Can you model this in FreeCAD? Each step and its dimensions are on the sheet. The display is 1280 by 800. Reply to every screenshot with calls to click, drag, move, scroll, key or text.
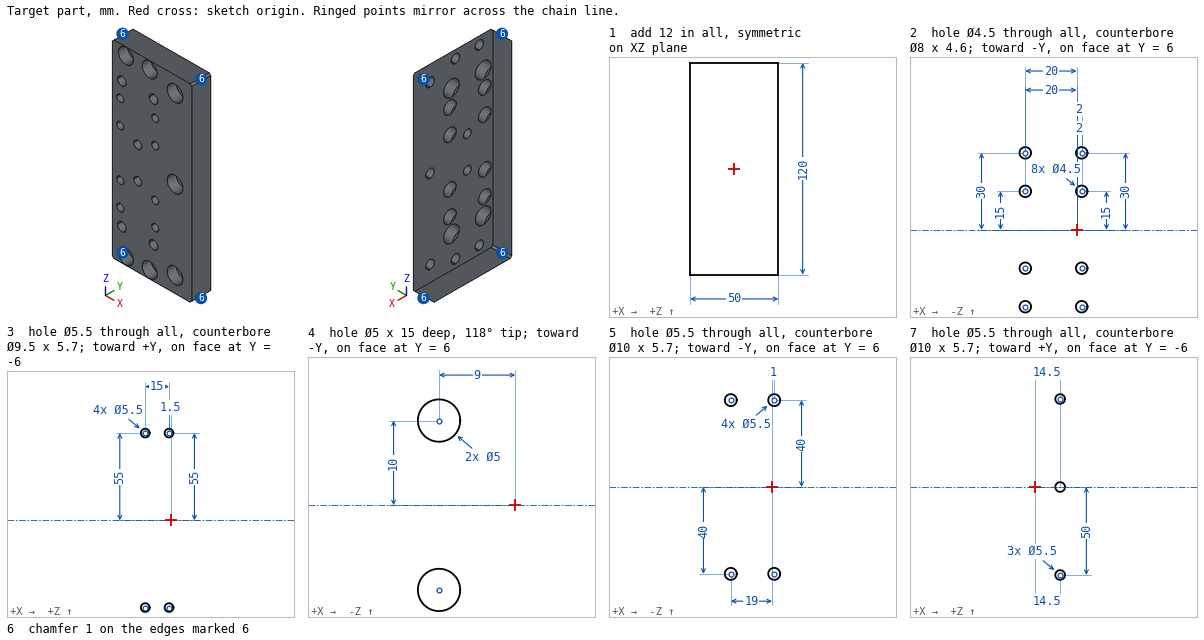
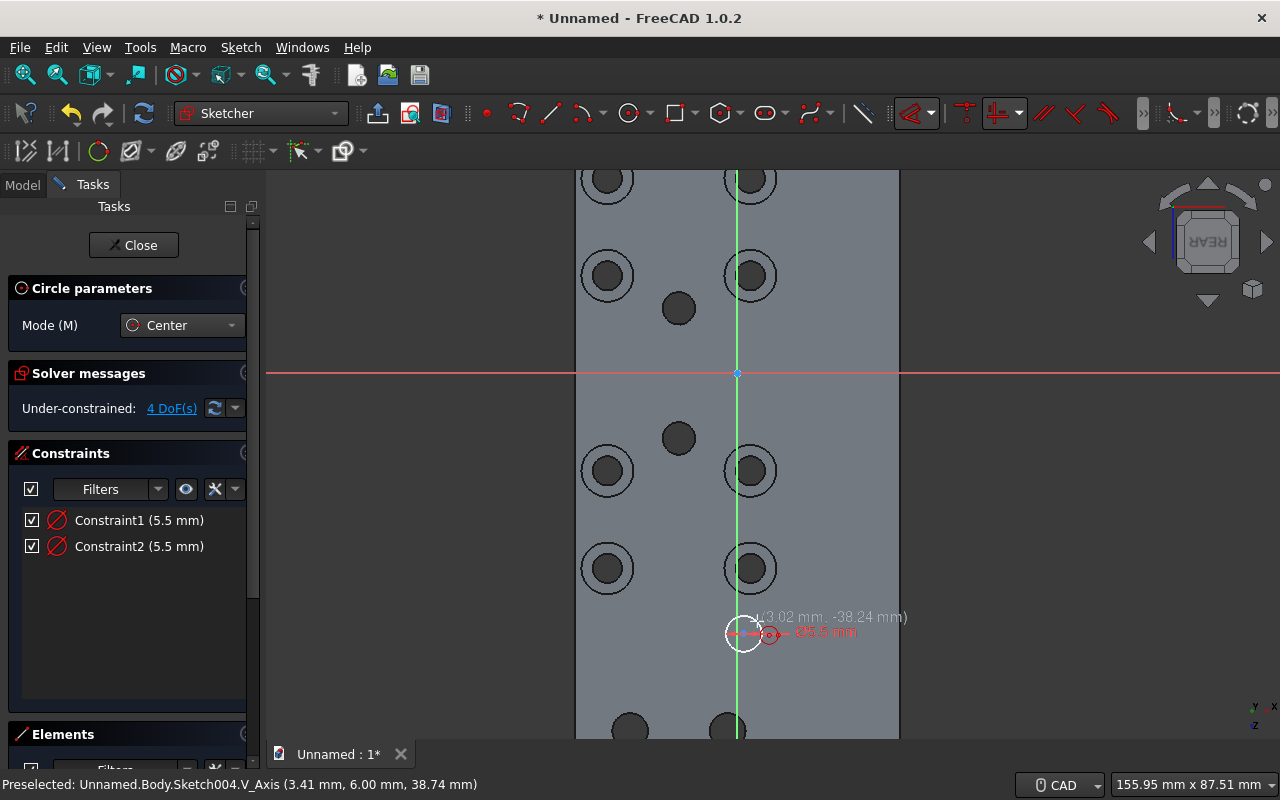
scroll(614, 633, up, 2)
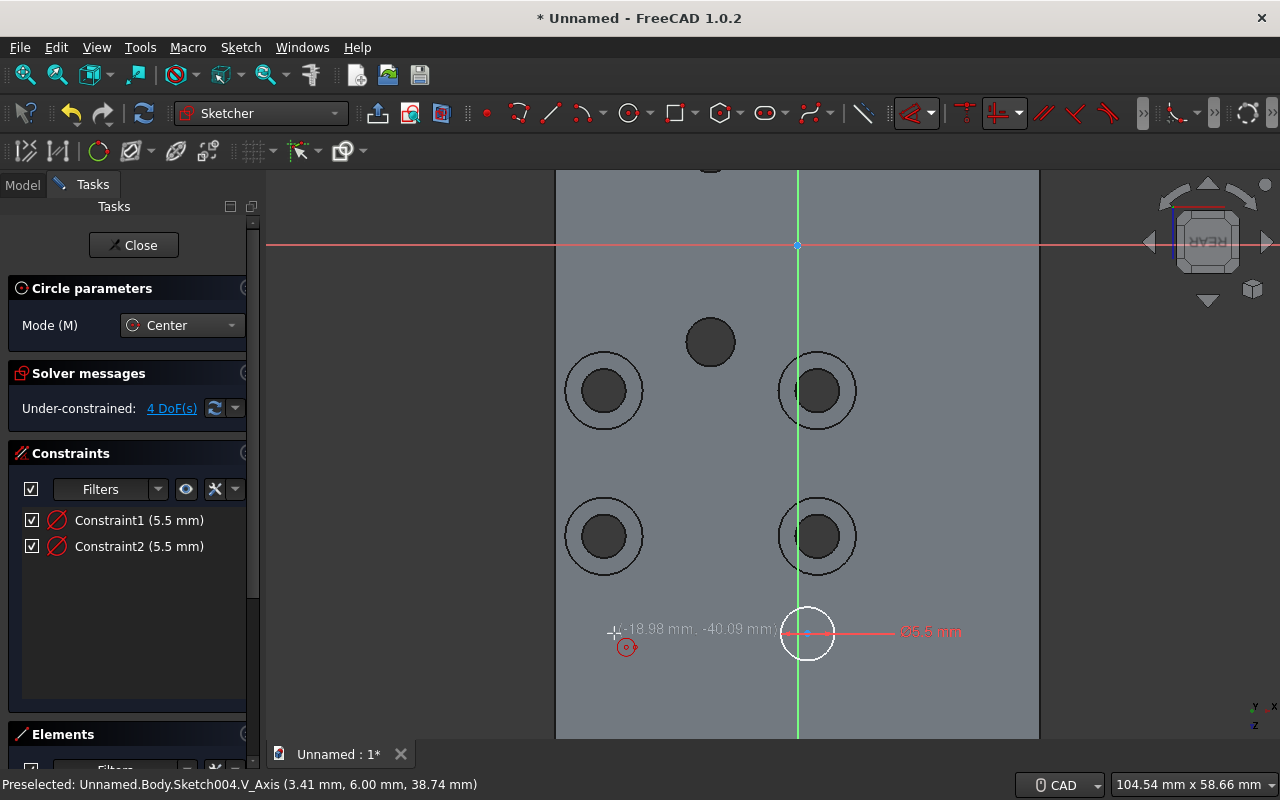
click(614, 633)
move(632, 614)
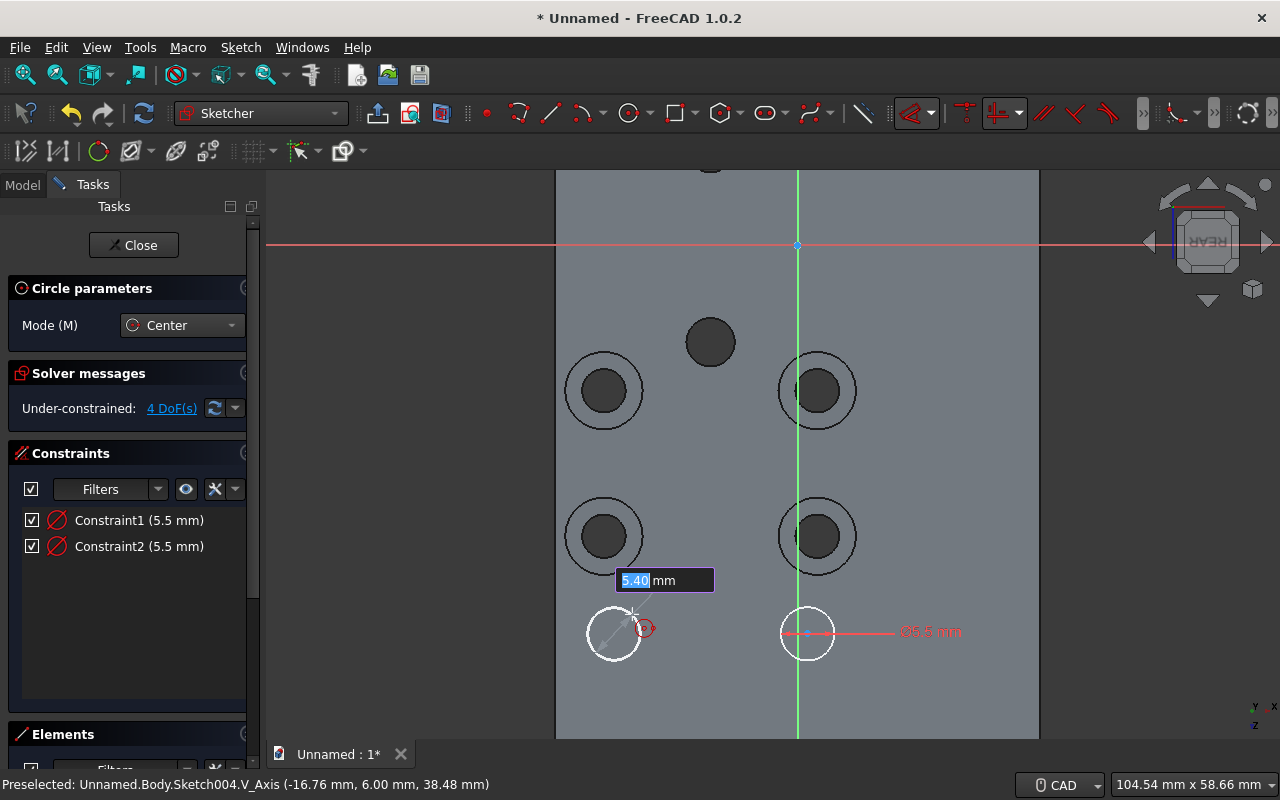
text(5.5)
key(Return)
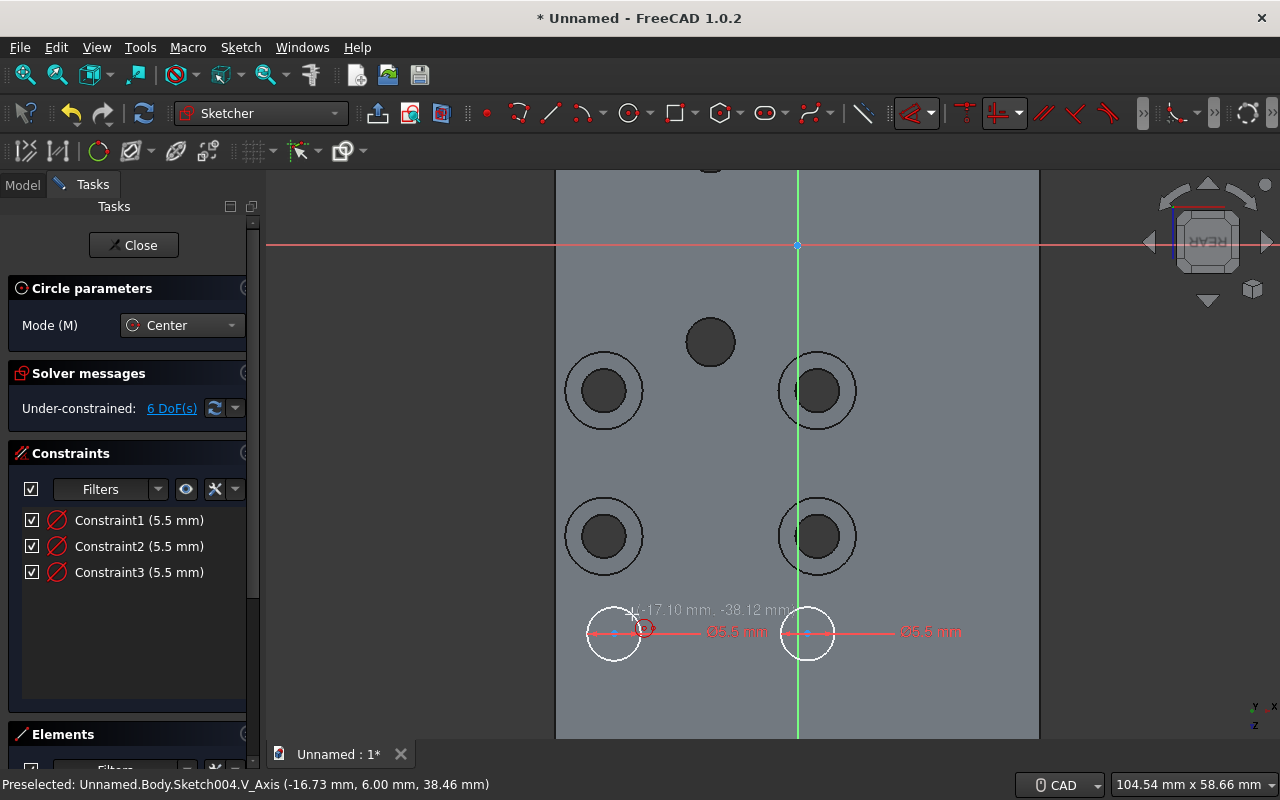
scroll(700, 625, down, 4)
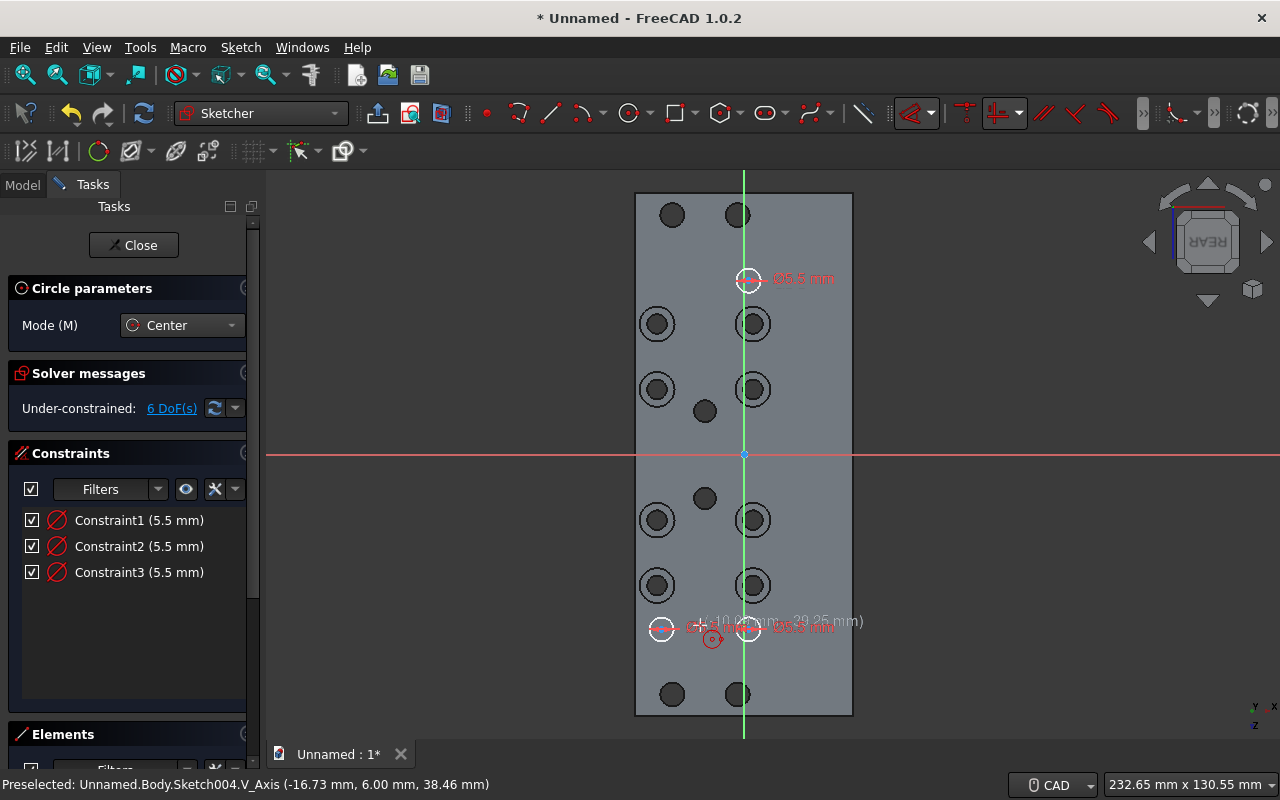
scroll(661, 280, up, 4)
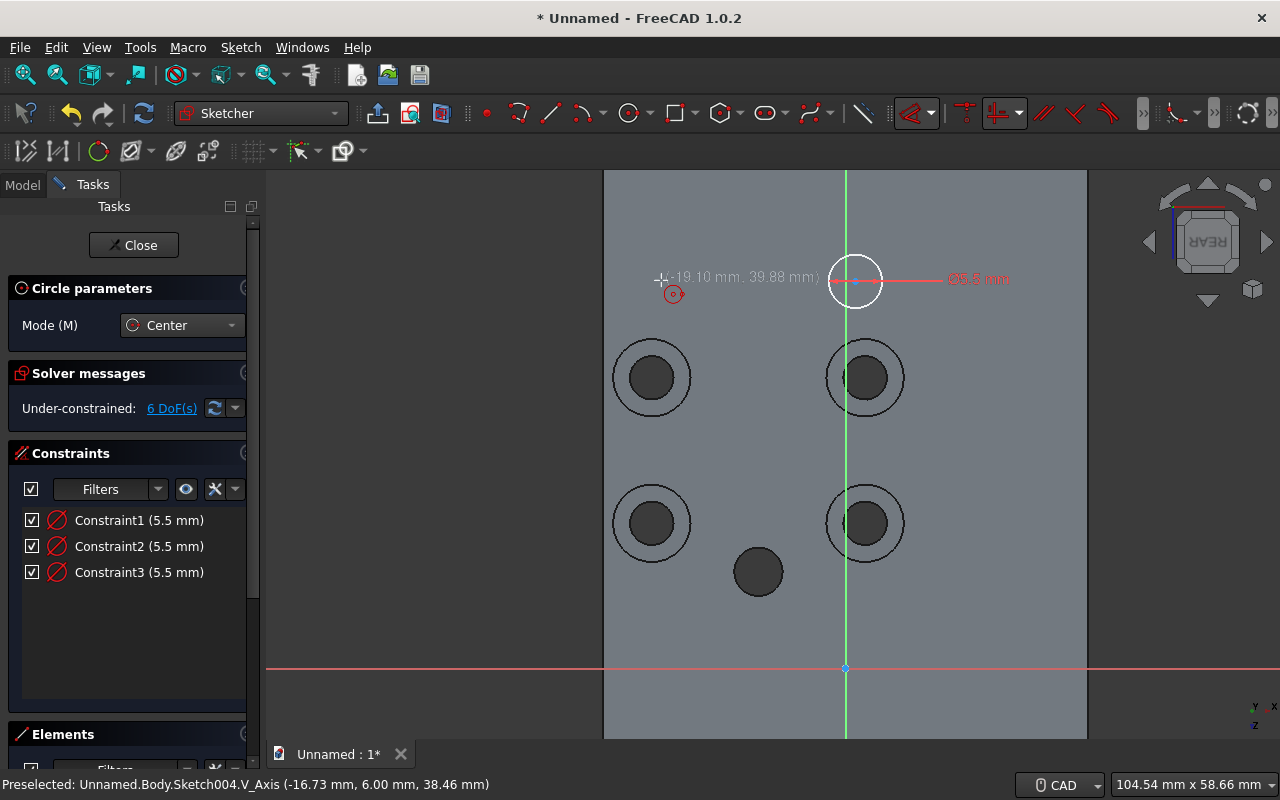
click(661, 281)
move(680, 262)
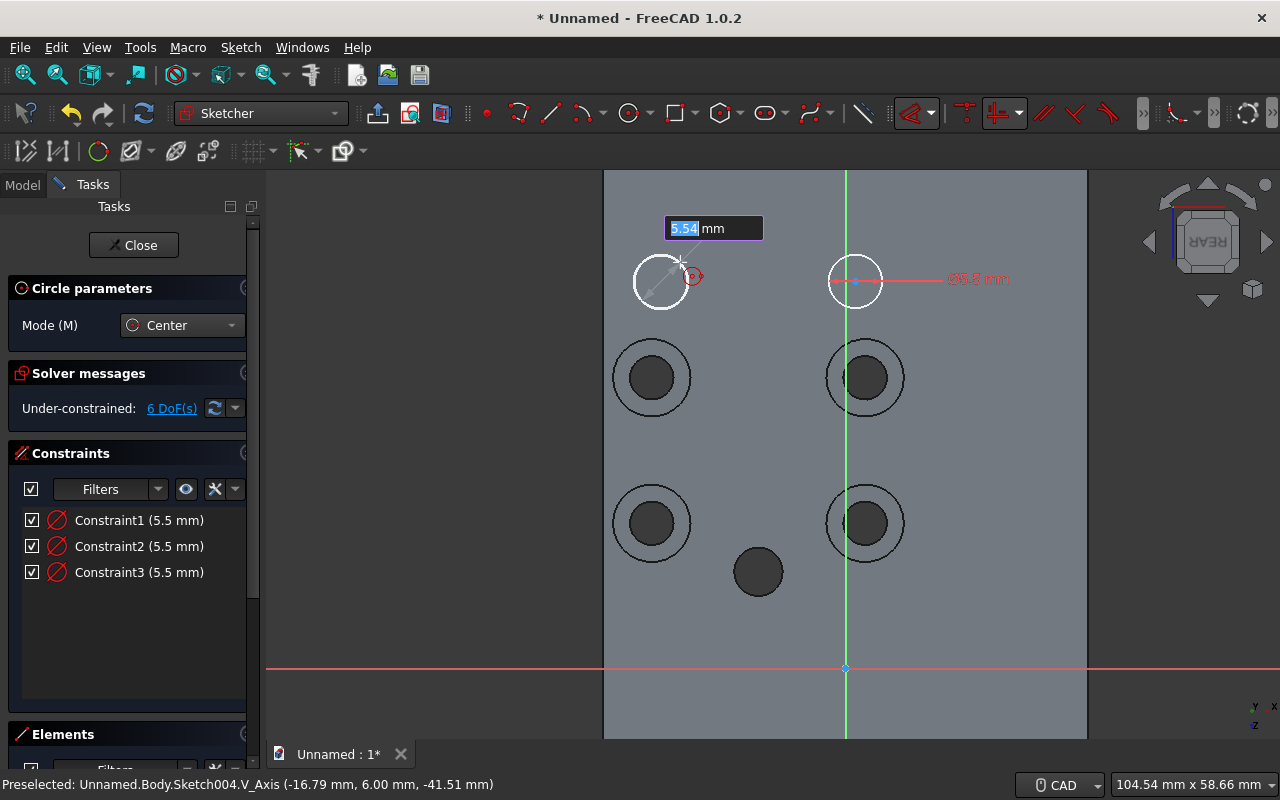
text(5.5)
key(Return)
key(Escape)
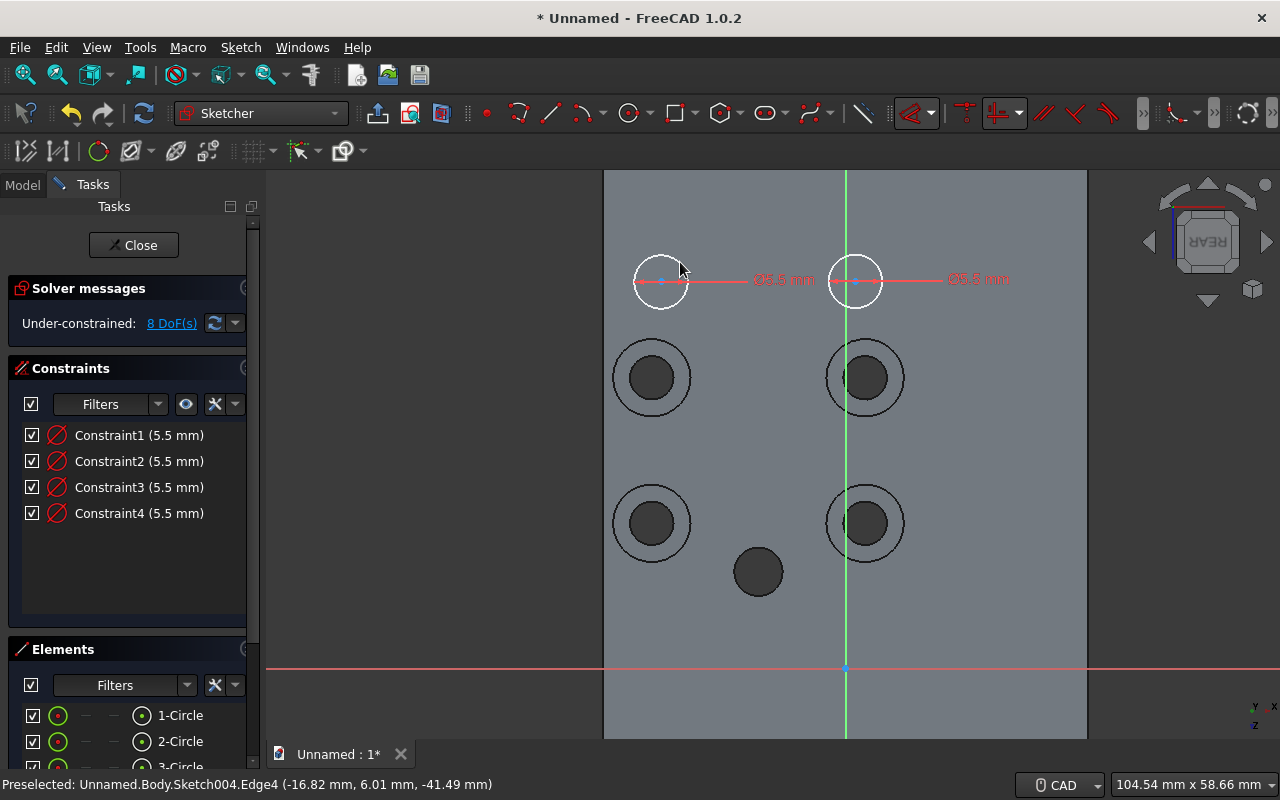
click(855, 281)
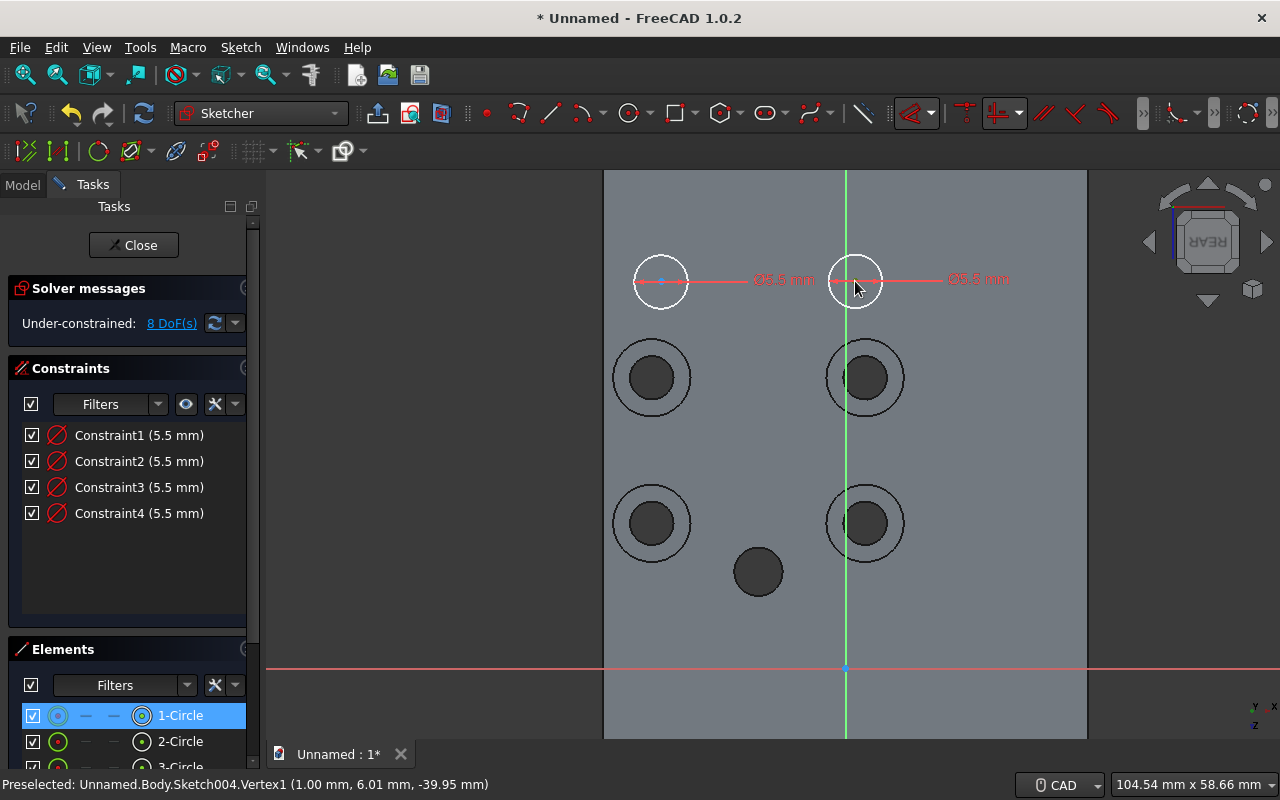
scroll(660, 280, down, 4)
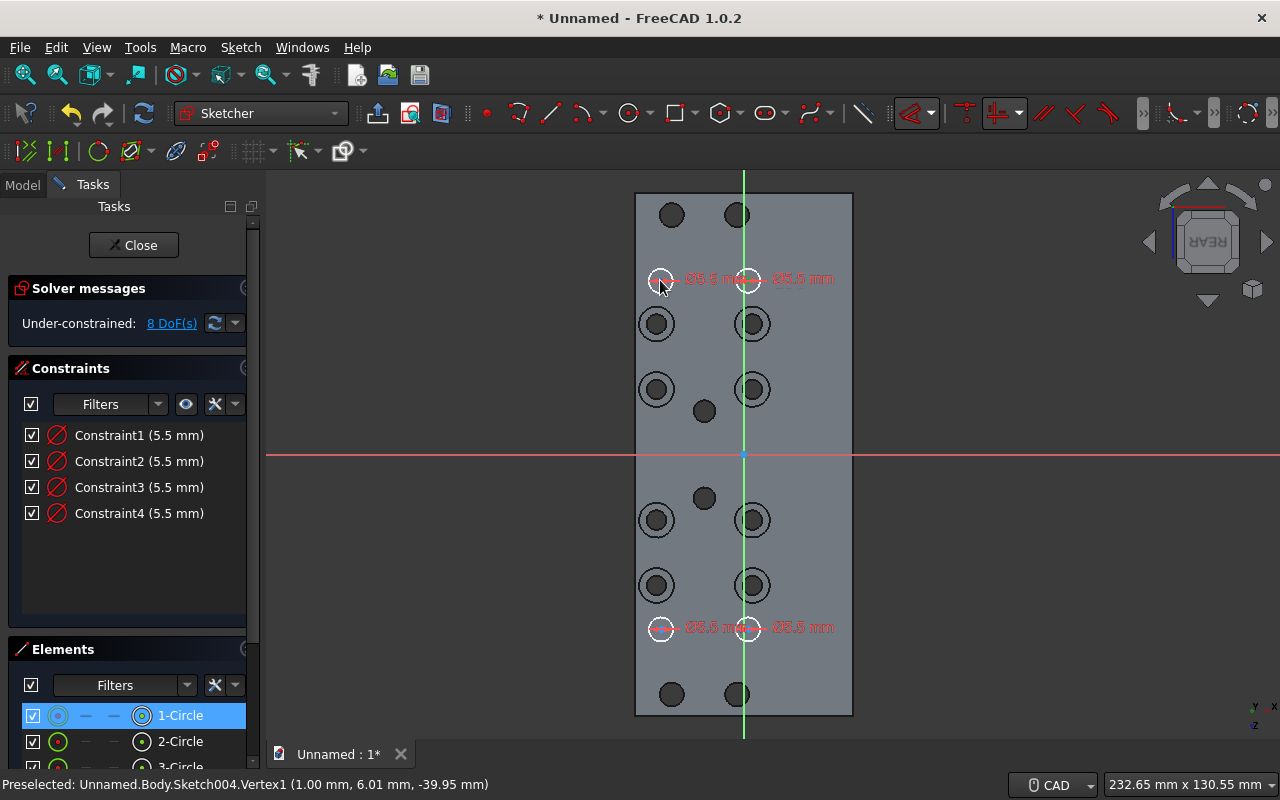
click(748, 629)